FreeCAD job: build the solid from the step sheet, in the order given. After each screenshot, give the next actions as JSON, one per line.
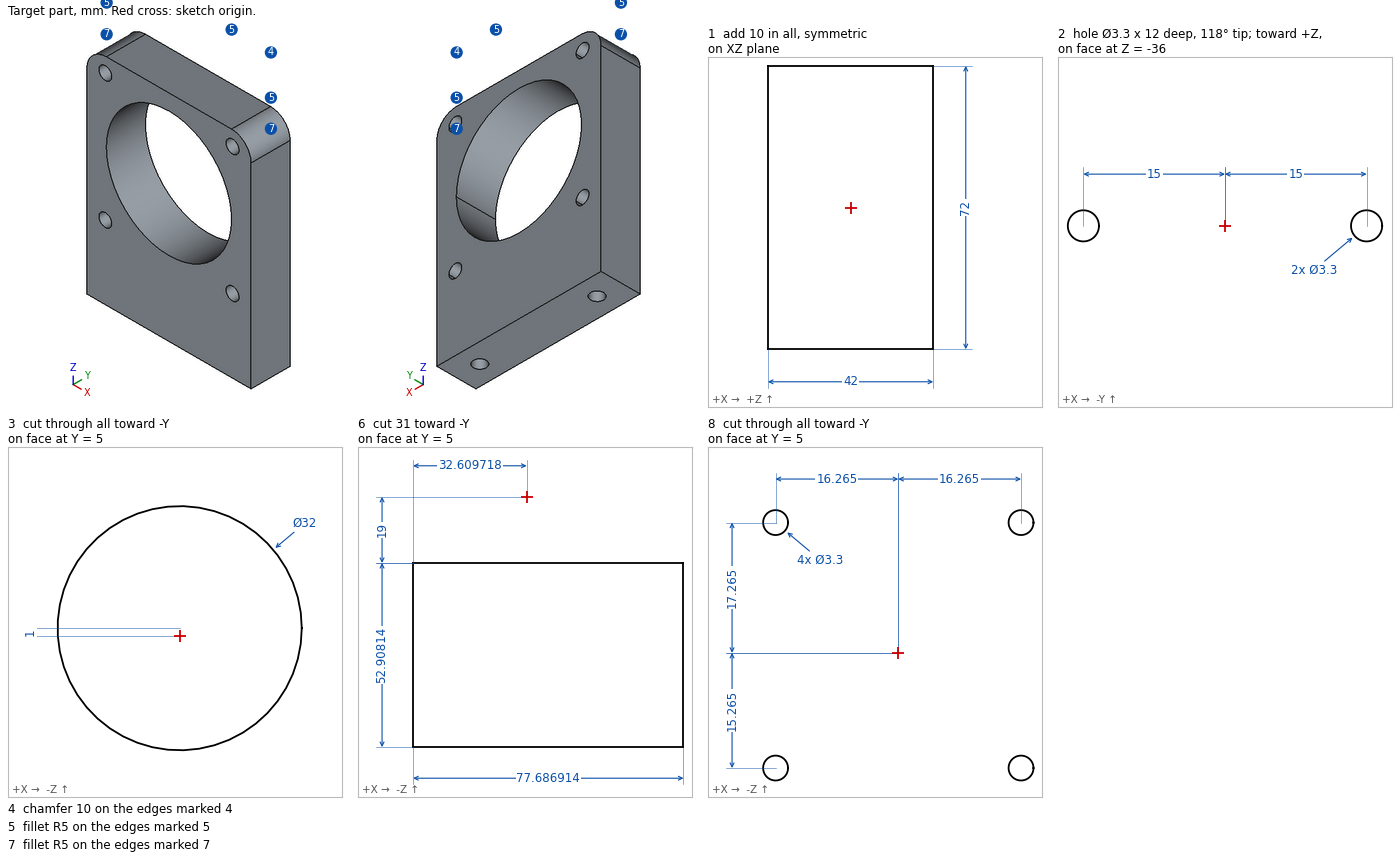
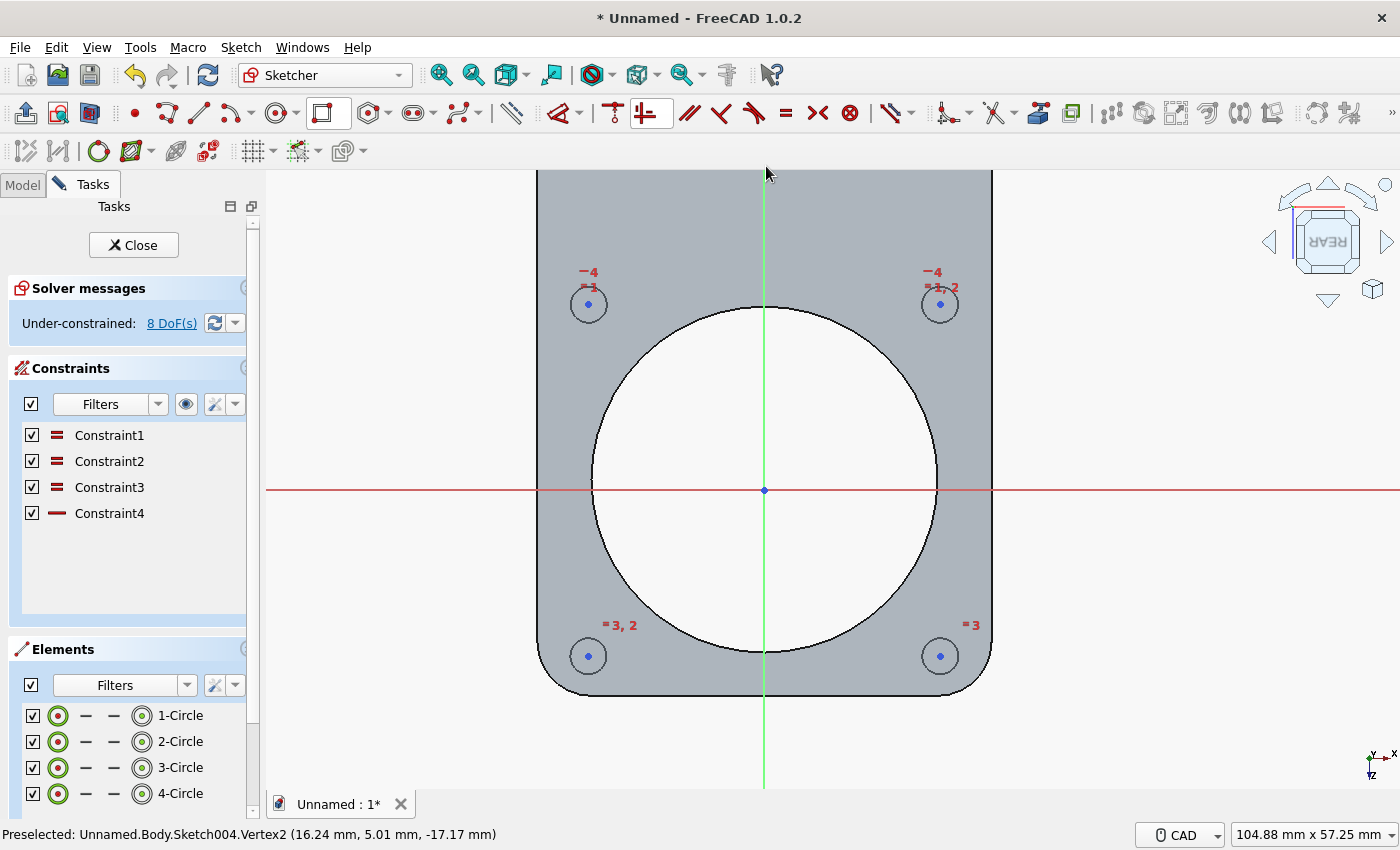
{"action": "left_click", "coordinate": [589, 305]}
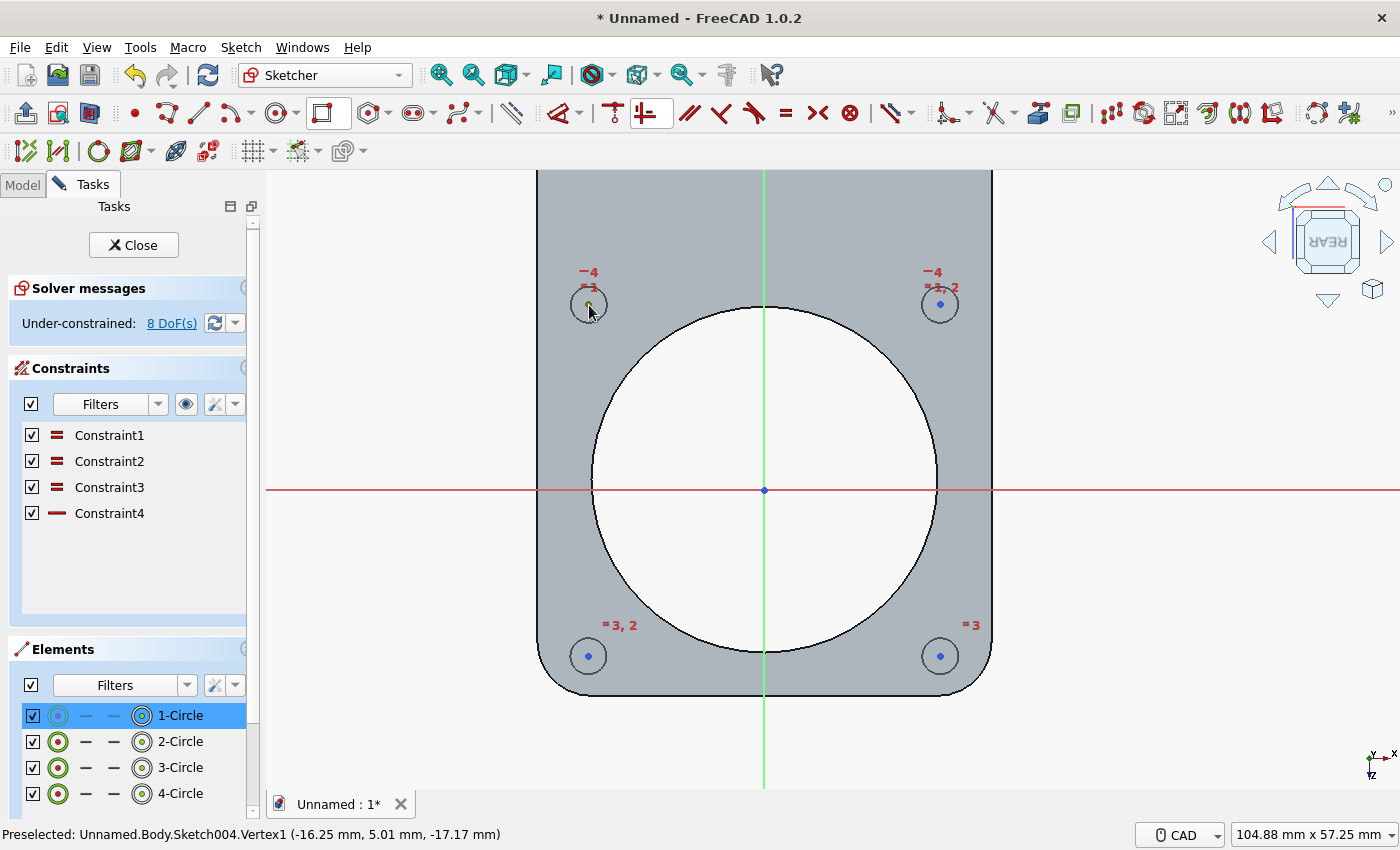
{"action": "left_click", "coordinate": [588, 656]}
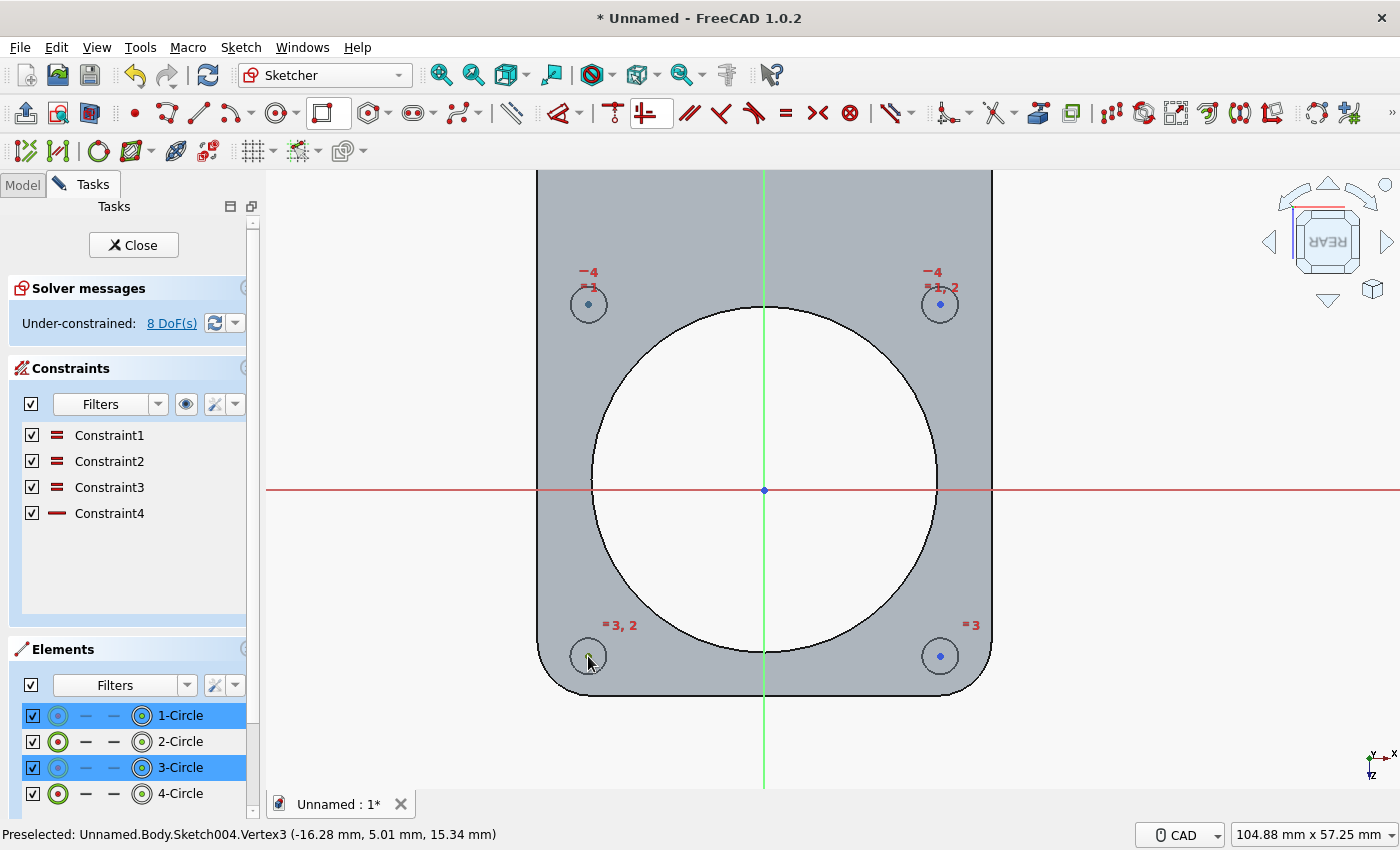
{"action": "key", "text": "v"}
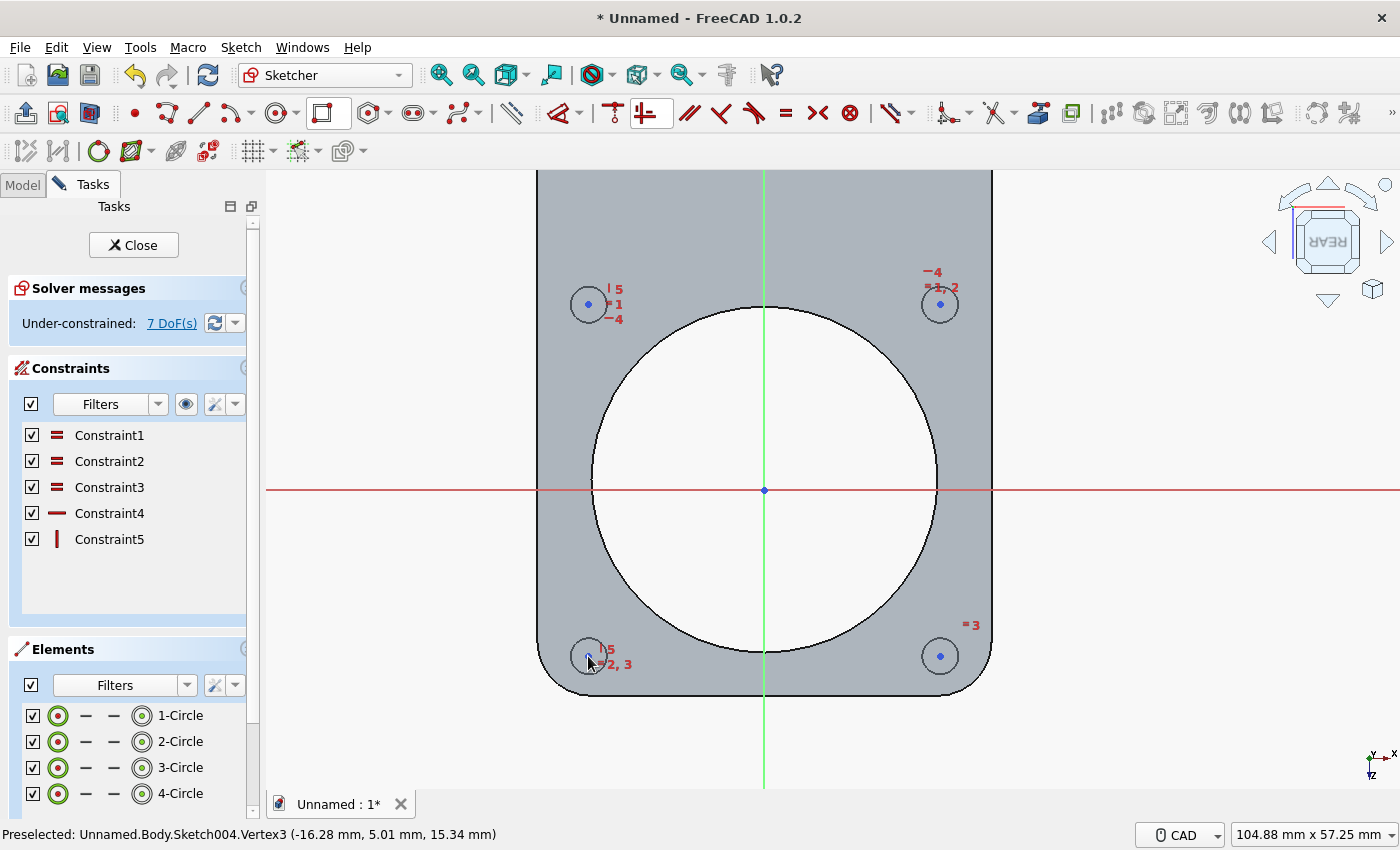
{"action": "left_click", "coordinate": [940, 305]}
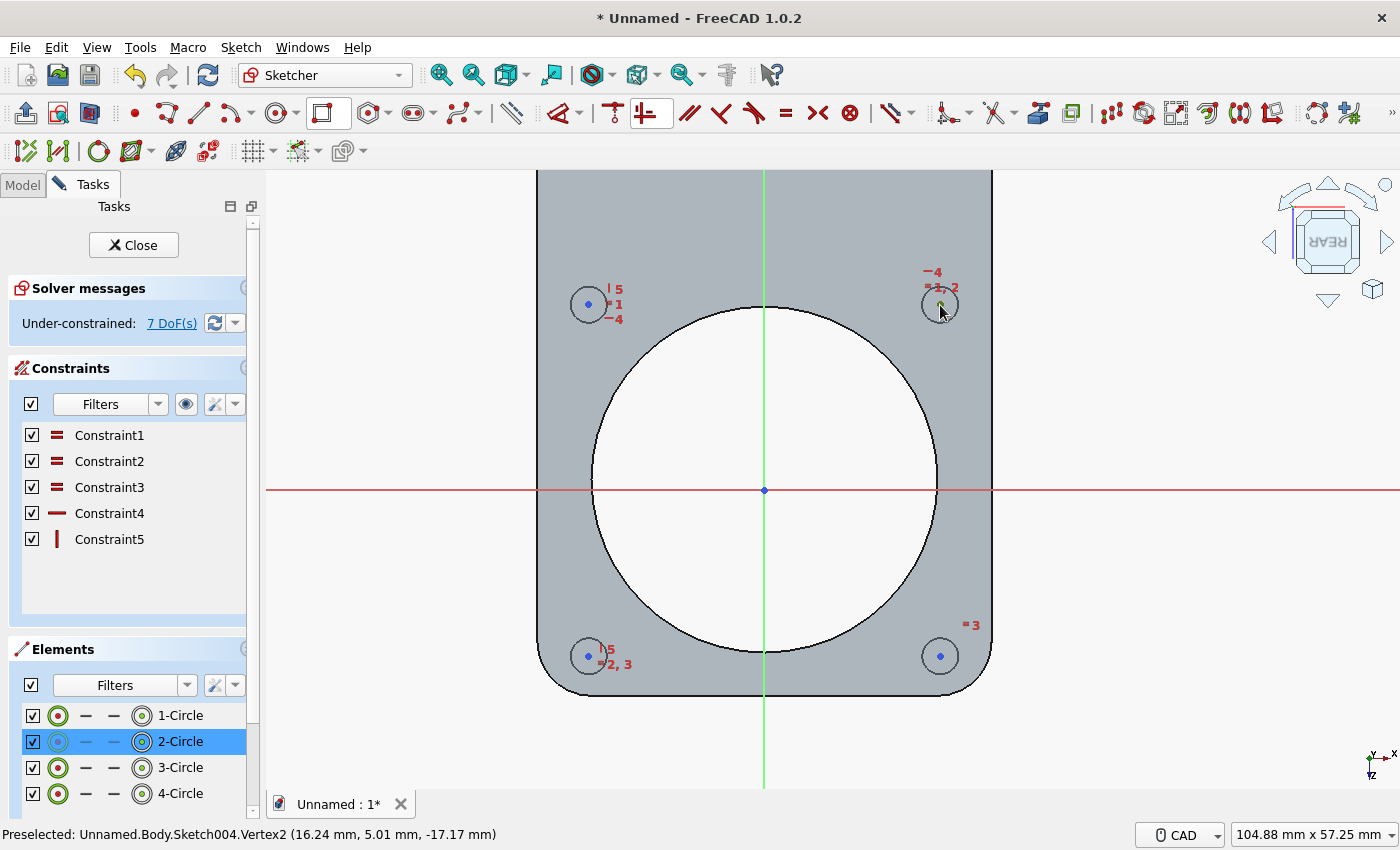
{"action": "left_click", "coordinate": [940, 656]}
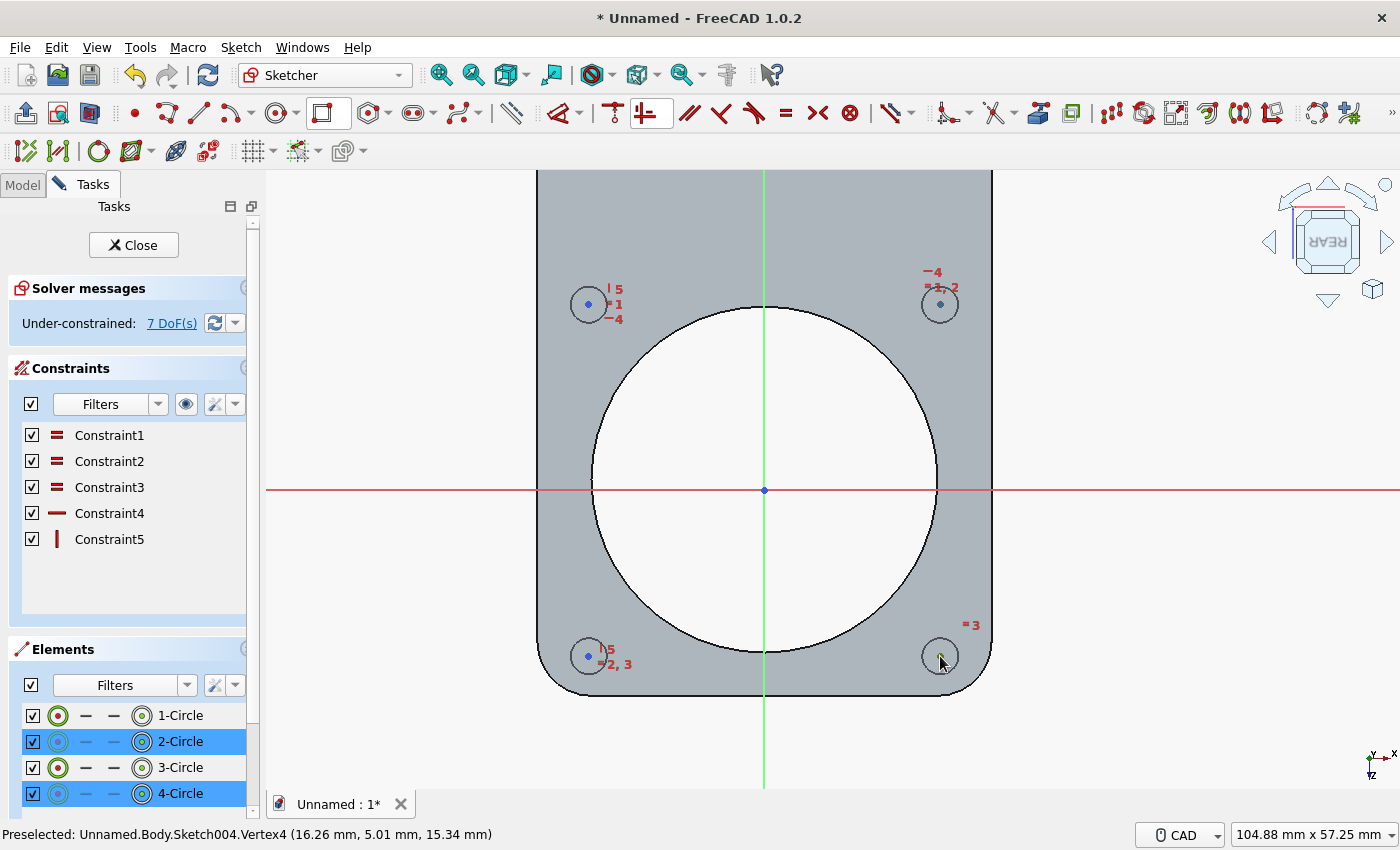
{"action": "left_click", "coordinate": [668, 114]}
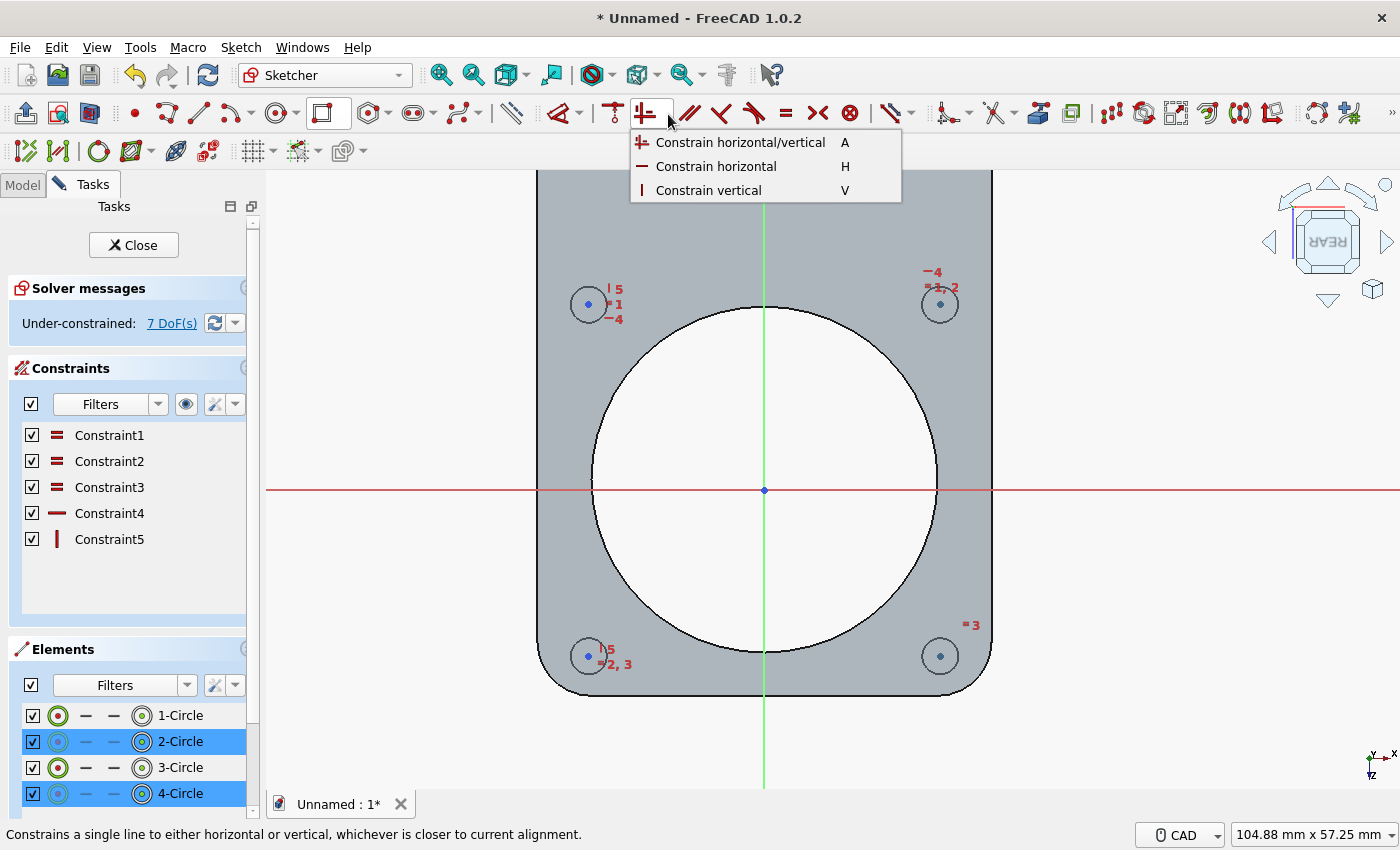
{"action": "left_click", "coordinate": [766, 190]}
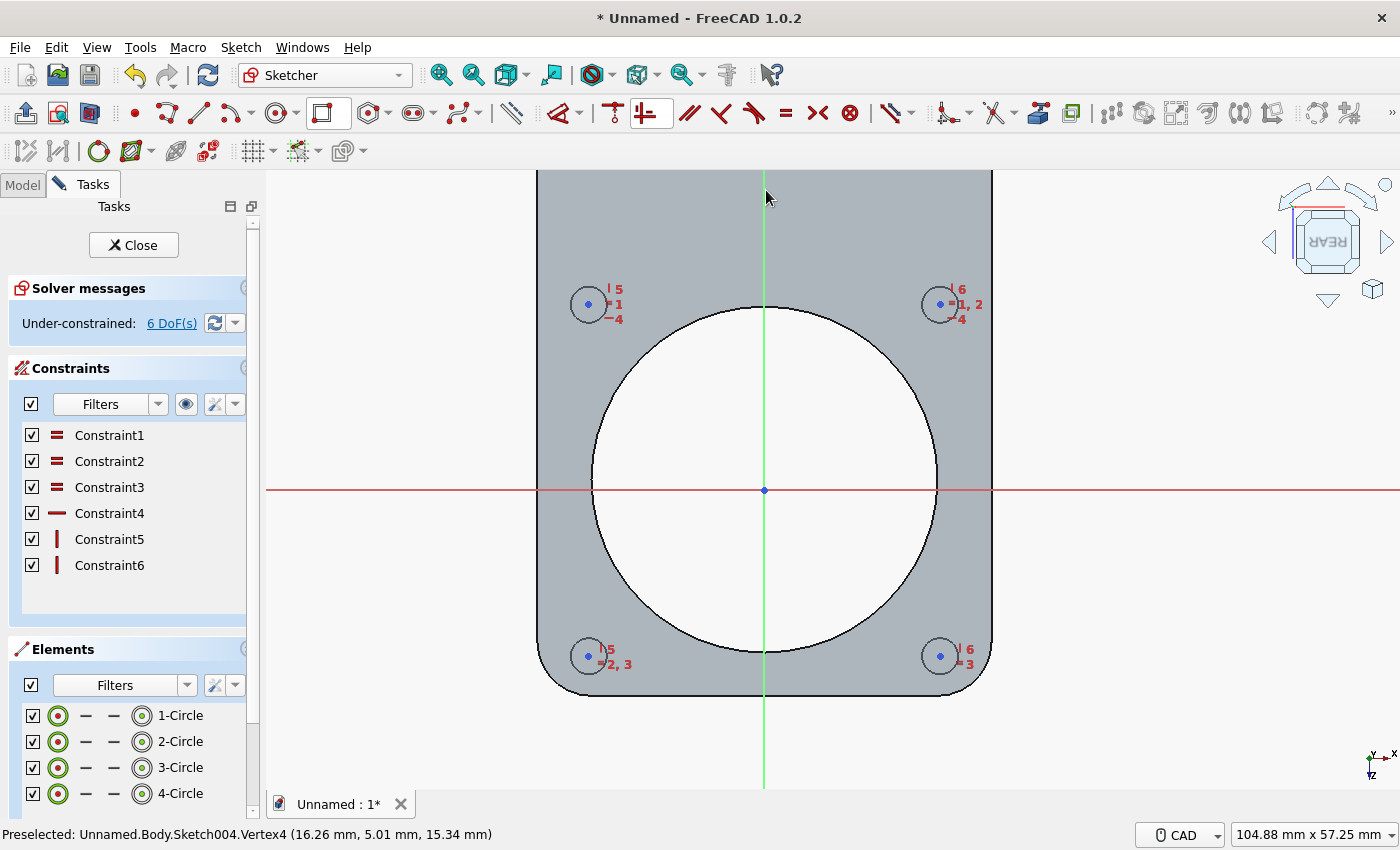
{"action": "left_click", "coordinate": [589, 656]}